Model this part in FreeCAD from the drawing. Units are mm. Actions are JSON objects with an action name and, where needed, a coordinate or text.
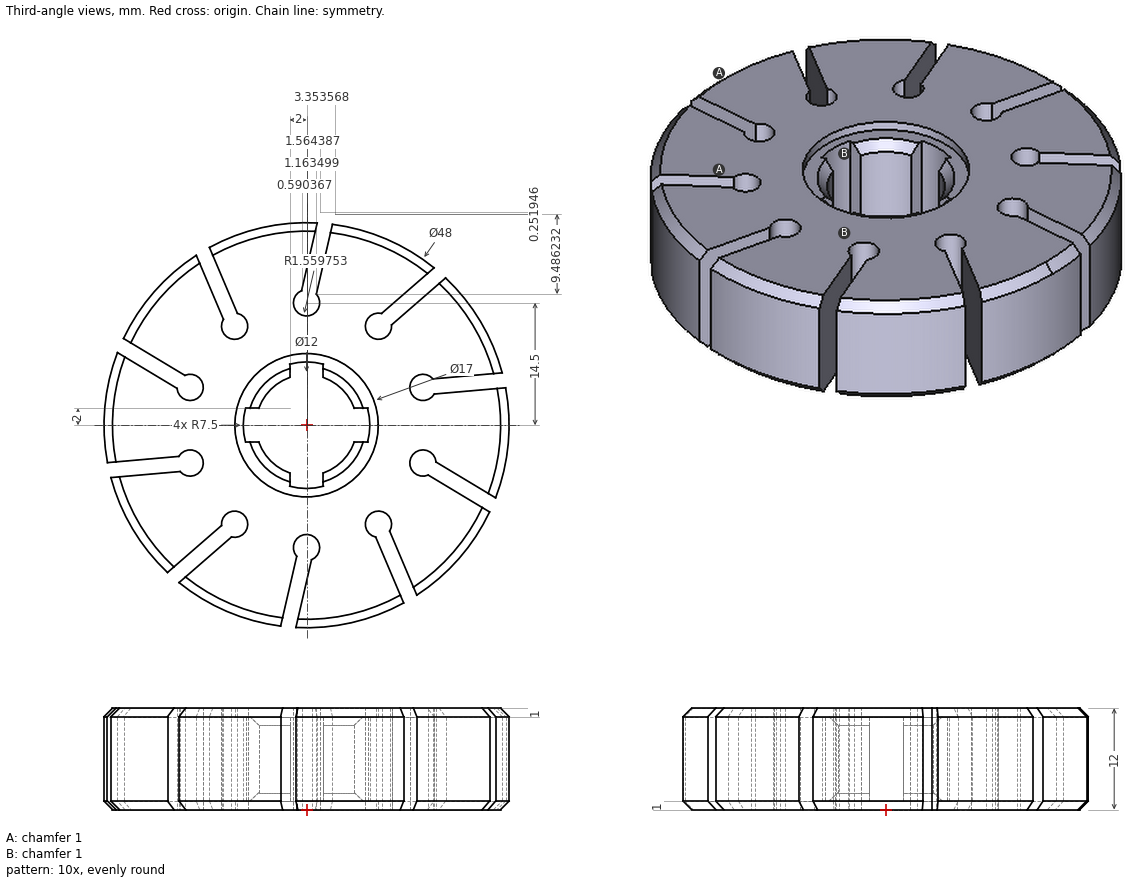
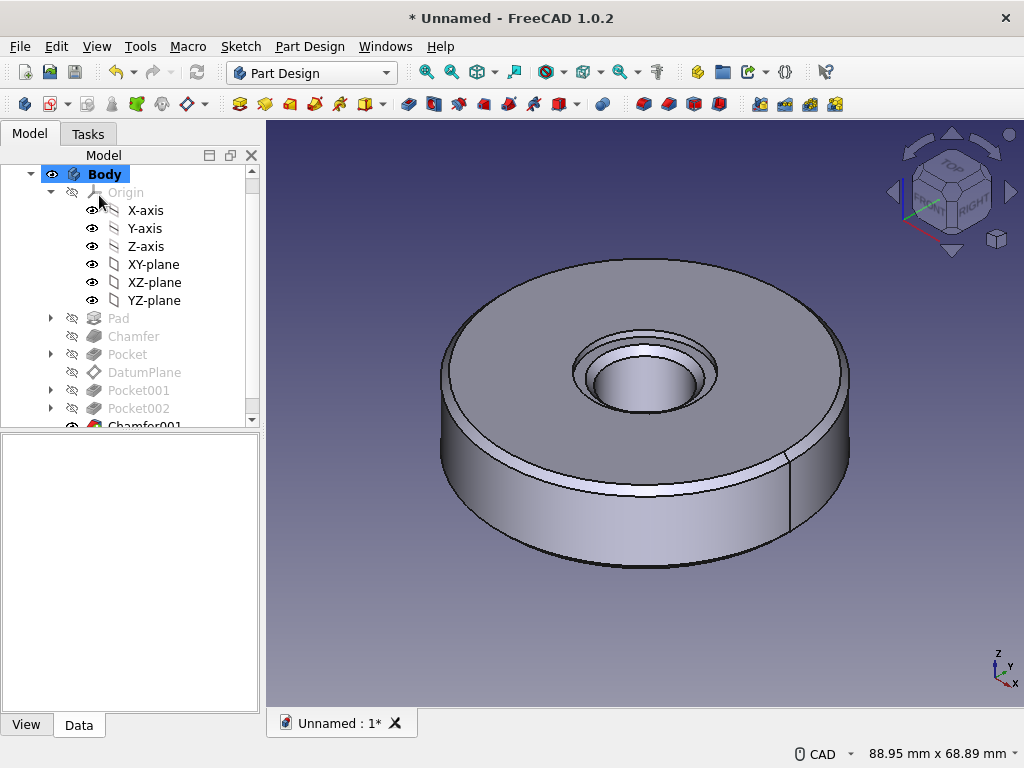
{"action": "scroll", "coordinate": [704, 361], "scroll_direction": "up", "scroll_amount": 4}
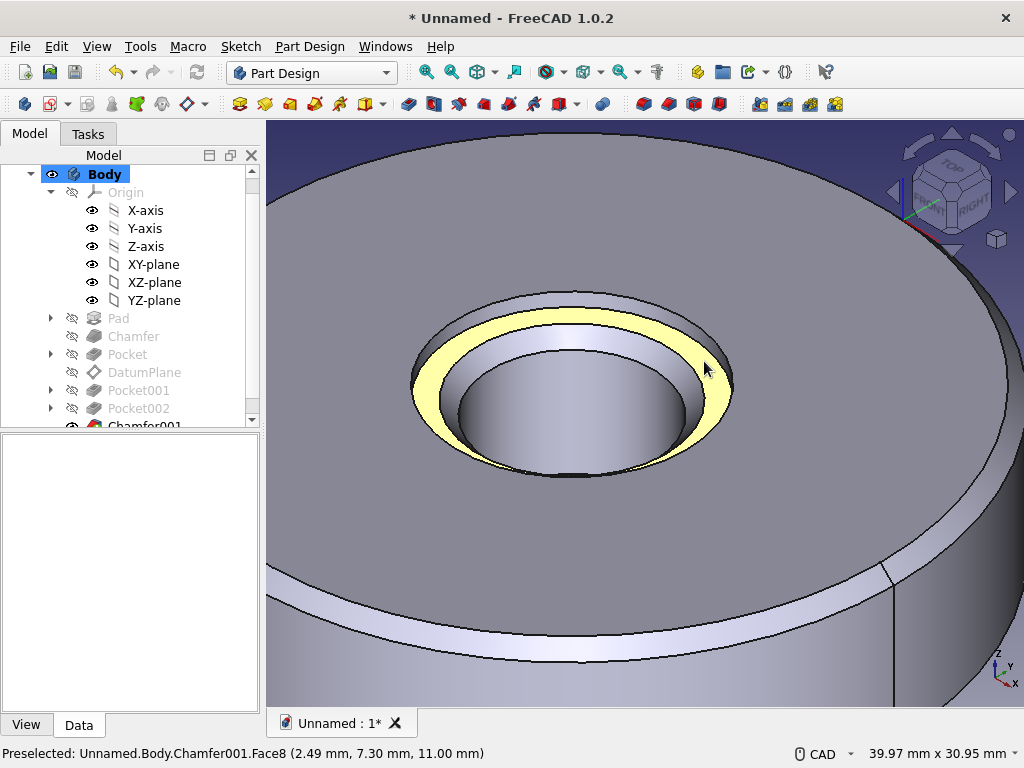
{"action": "left_click", "coordinate": [702, 361]}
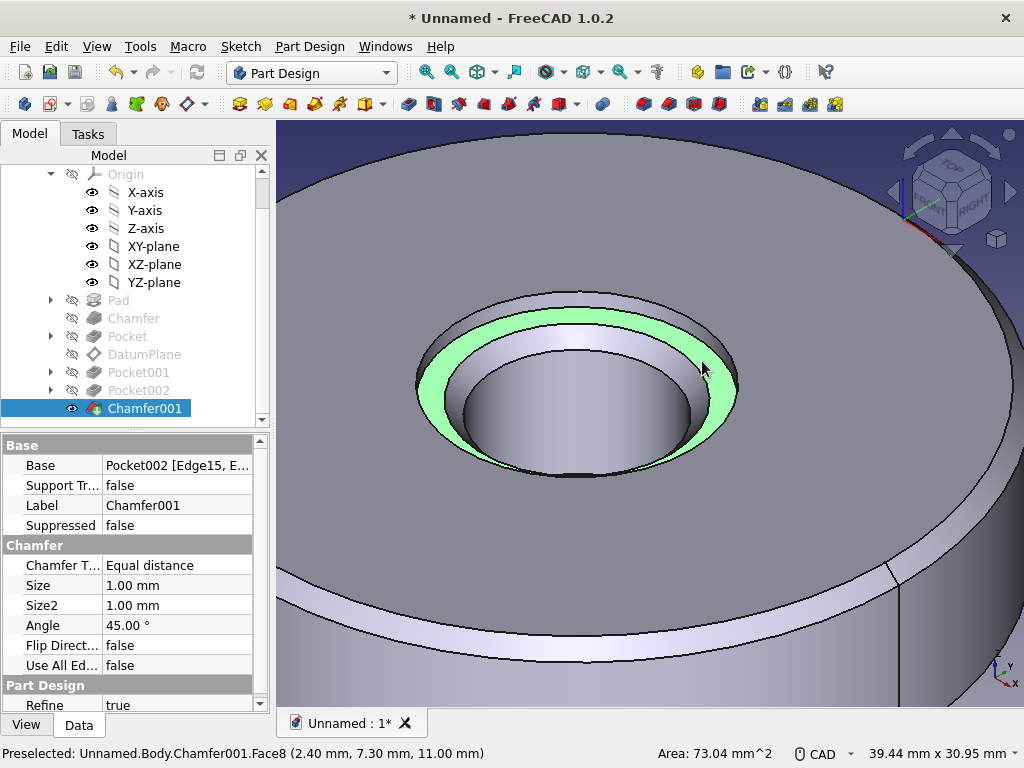
{"action": "left_click", "coordinate": [50, 104]}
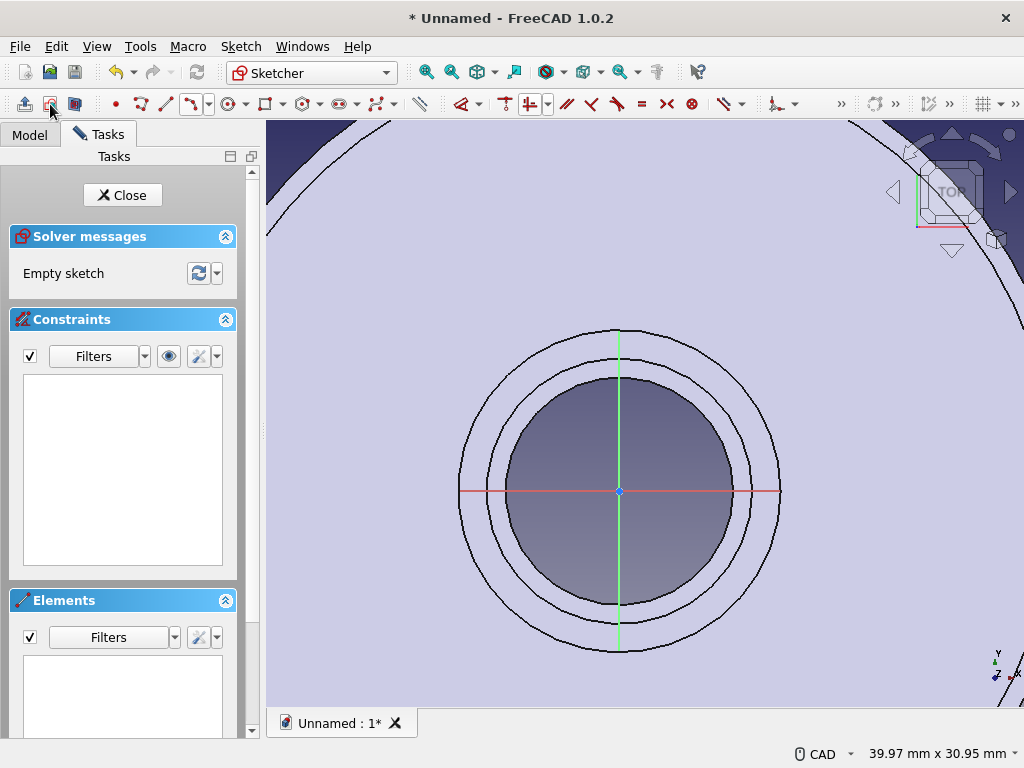
{"action": "left_click", "coordinate": [75, 104]}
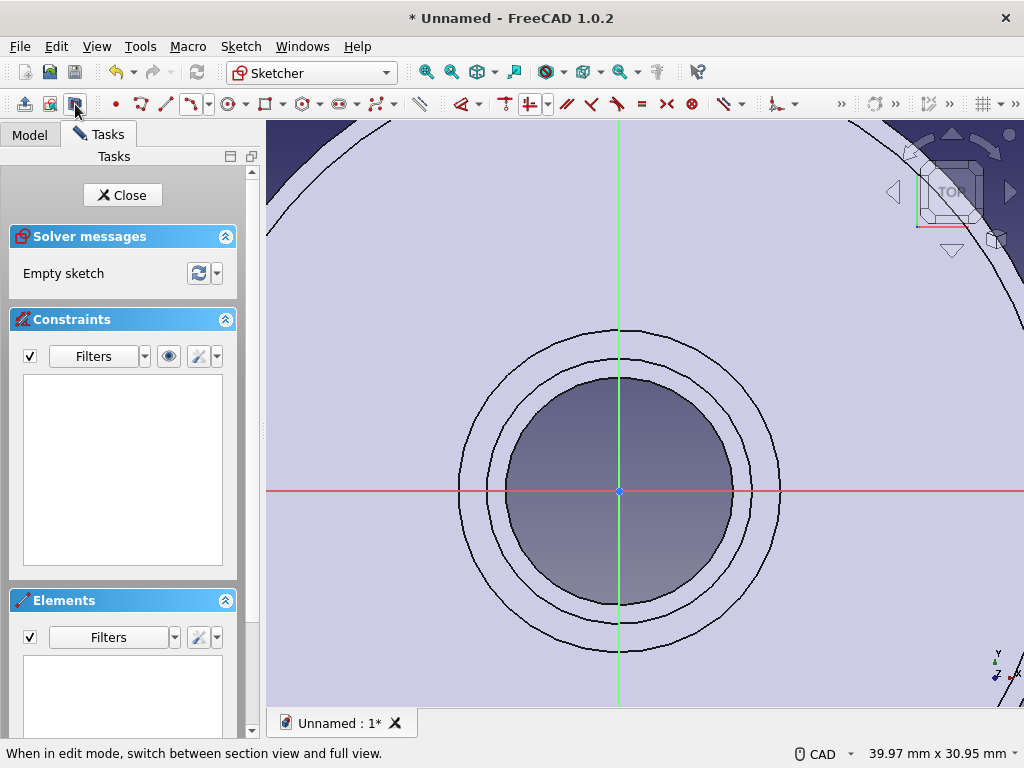
{"action": "left_click", "coordinate": [141, 104]}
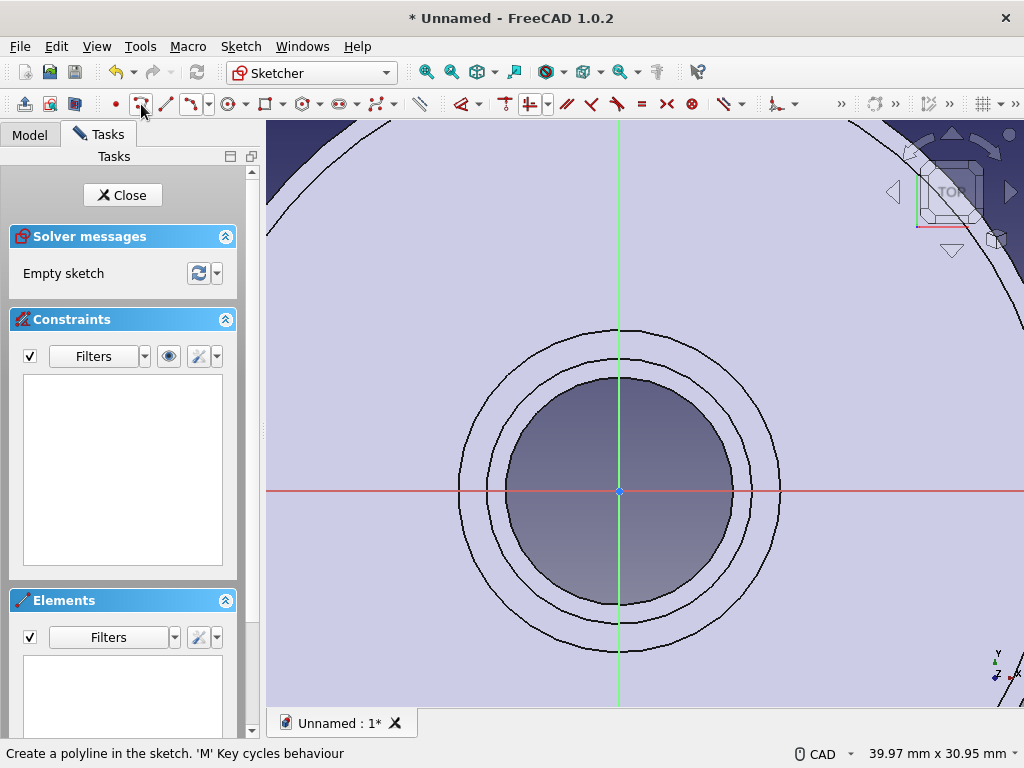
{"action": "left_click", "coordinate": [582, 354]}
{"action": "left_click", "coordinate": [582, 453]}
{"action": "left_click", "coordinate": [482, 453]}
{"action": "right_click", "coordinate": [482, 453]}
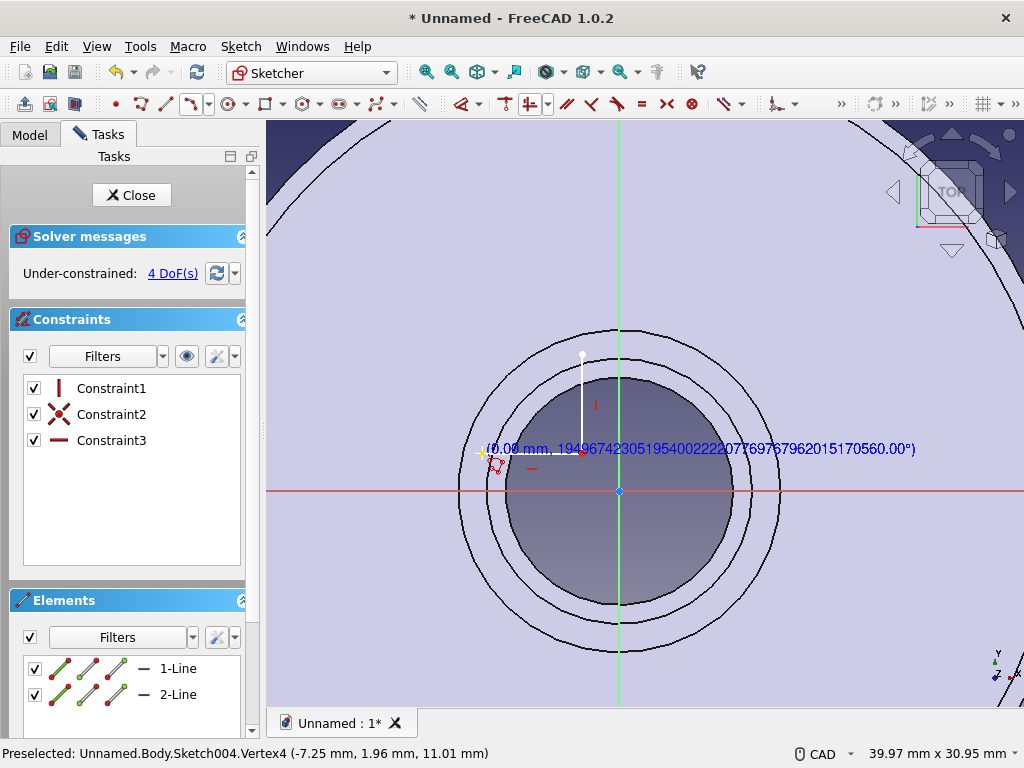
{"action": "left_click", "coordinate": [482, 529]}
{"action": "left_click", "coordinate": [582, 529]}
{"action": "left_click", "coordinate": [582, 628]}
{"action": "right_click", "coordinate": [582, 628]}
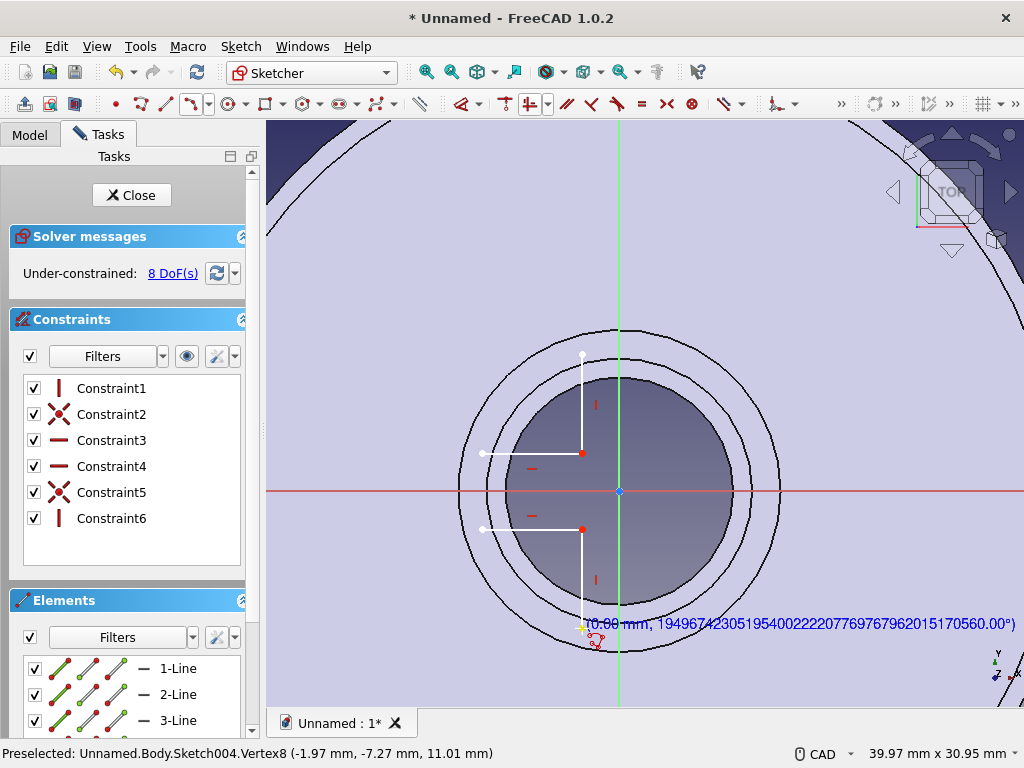
{"action": "left_click", "coordinate": [657, 628]}
{"action": "left_click", "coordinate": [657, 529]}
{"action": "left_click", "coordinate": [757, 529]}
{"action": "right_click", "coordinate": [757, 529]}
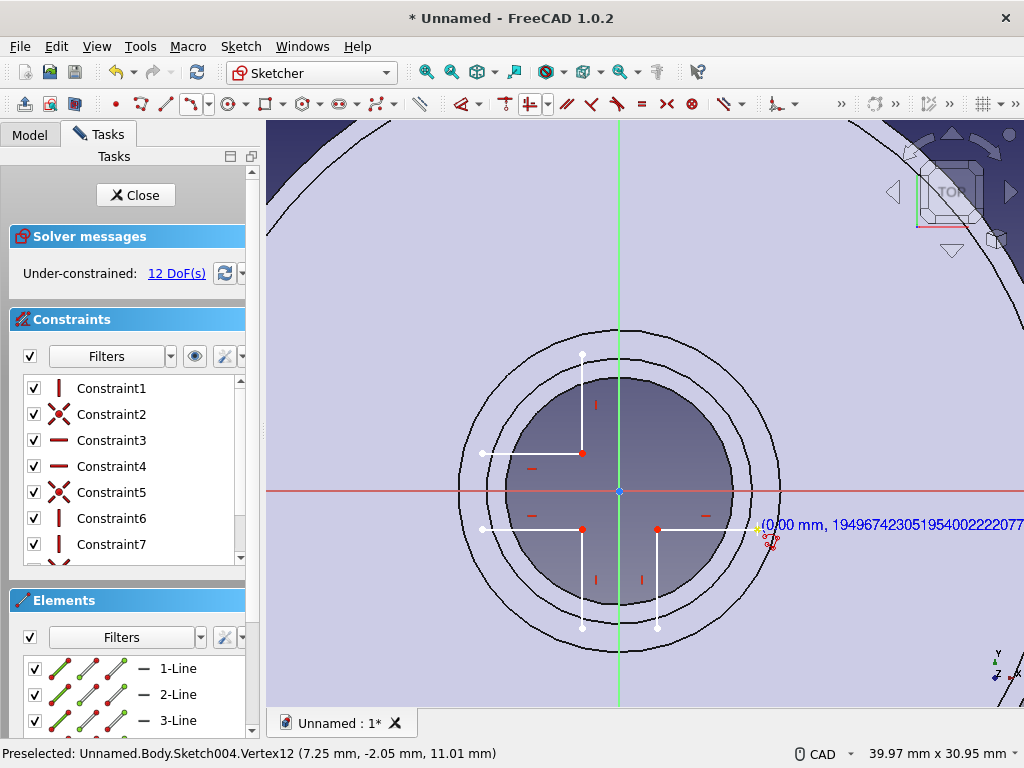
{"action": "left_click", "coordinate": [757, 453]}
{"action": "left_click", "coordinate": [657, 453]}
{"action": "left_click", "coordinate": [657, 354]}
{"action": "right_click", "coordinate": [657, 354]}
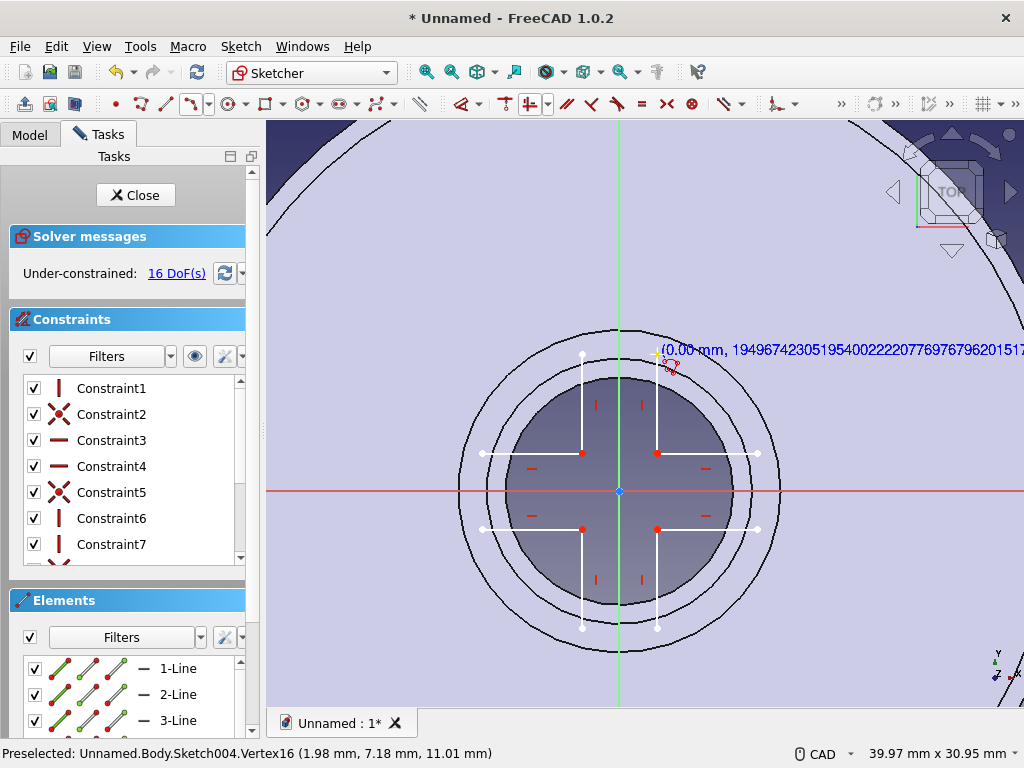
{"action": "left_click", "coordinate": [190, 104]}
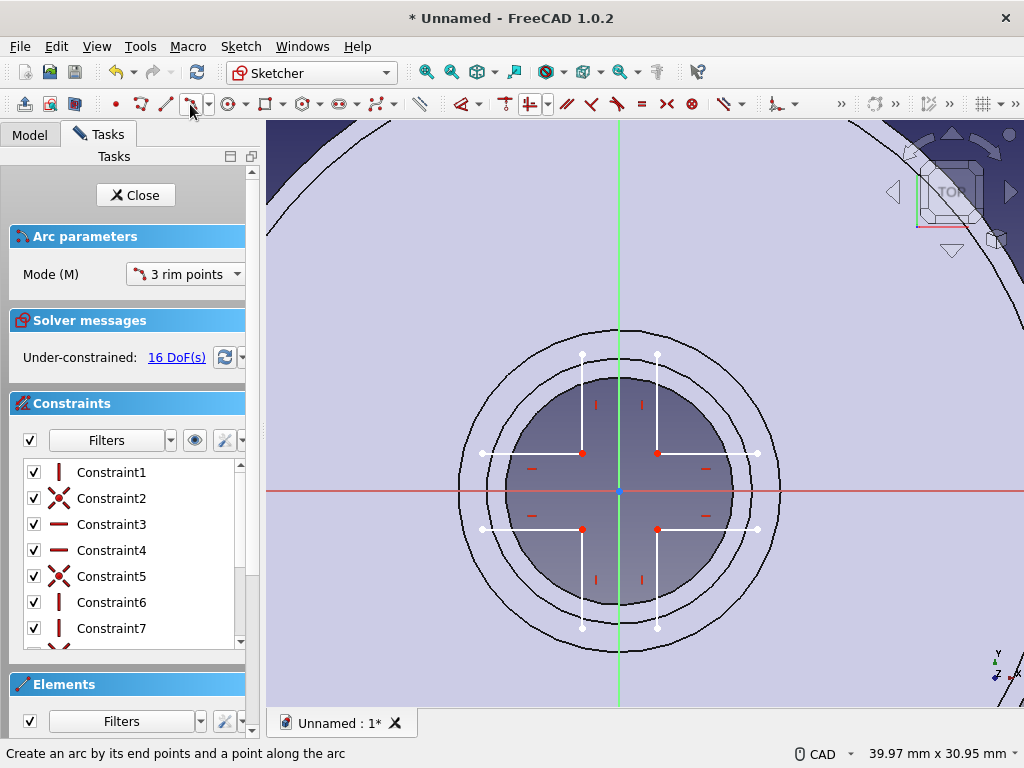
{"action": "left_click", "coordinate": [482, 454]}
{"action": "left_click", "coordinate": [482, 530]}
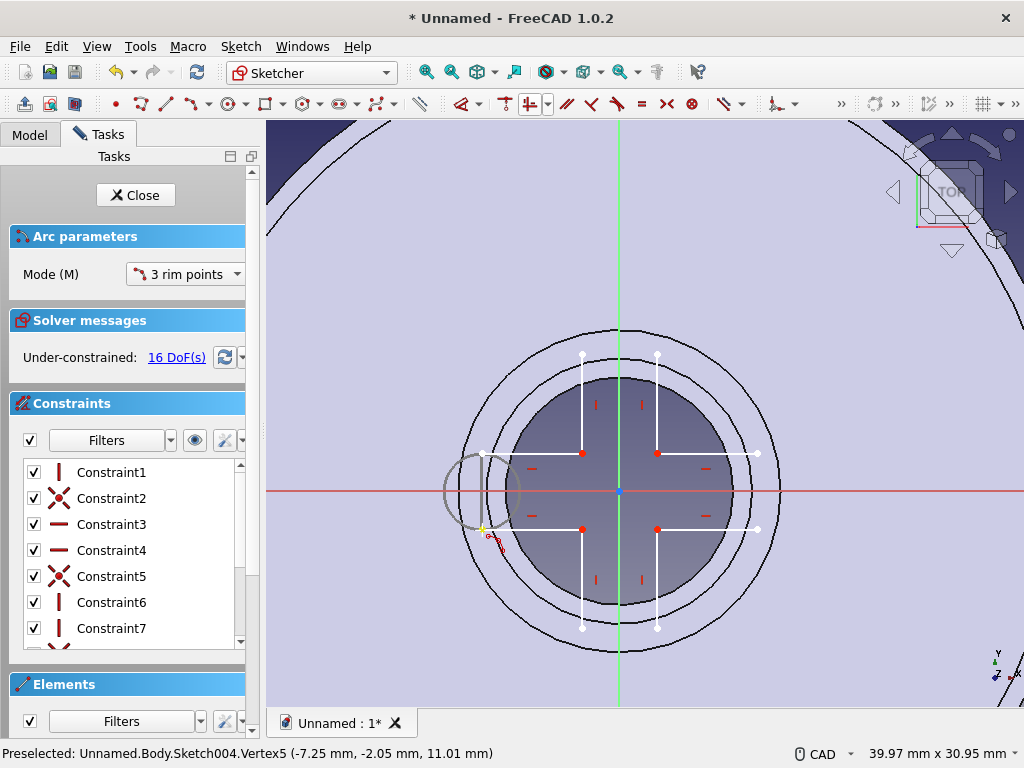
{"action": "scroll", "coordinate": [477, 484], "scroll_direction": "up", "scroll_amount": 6}